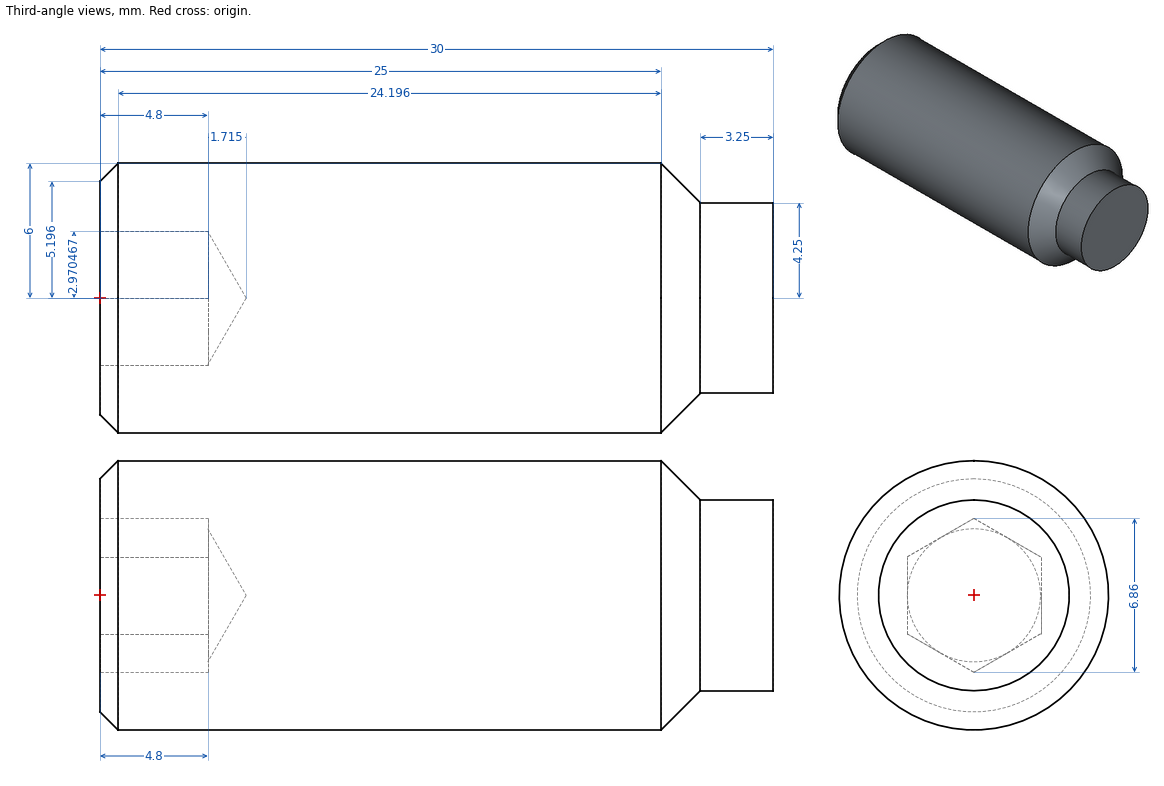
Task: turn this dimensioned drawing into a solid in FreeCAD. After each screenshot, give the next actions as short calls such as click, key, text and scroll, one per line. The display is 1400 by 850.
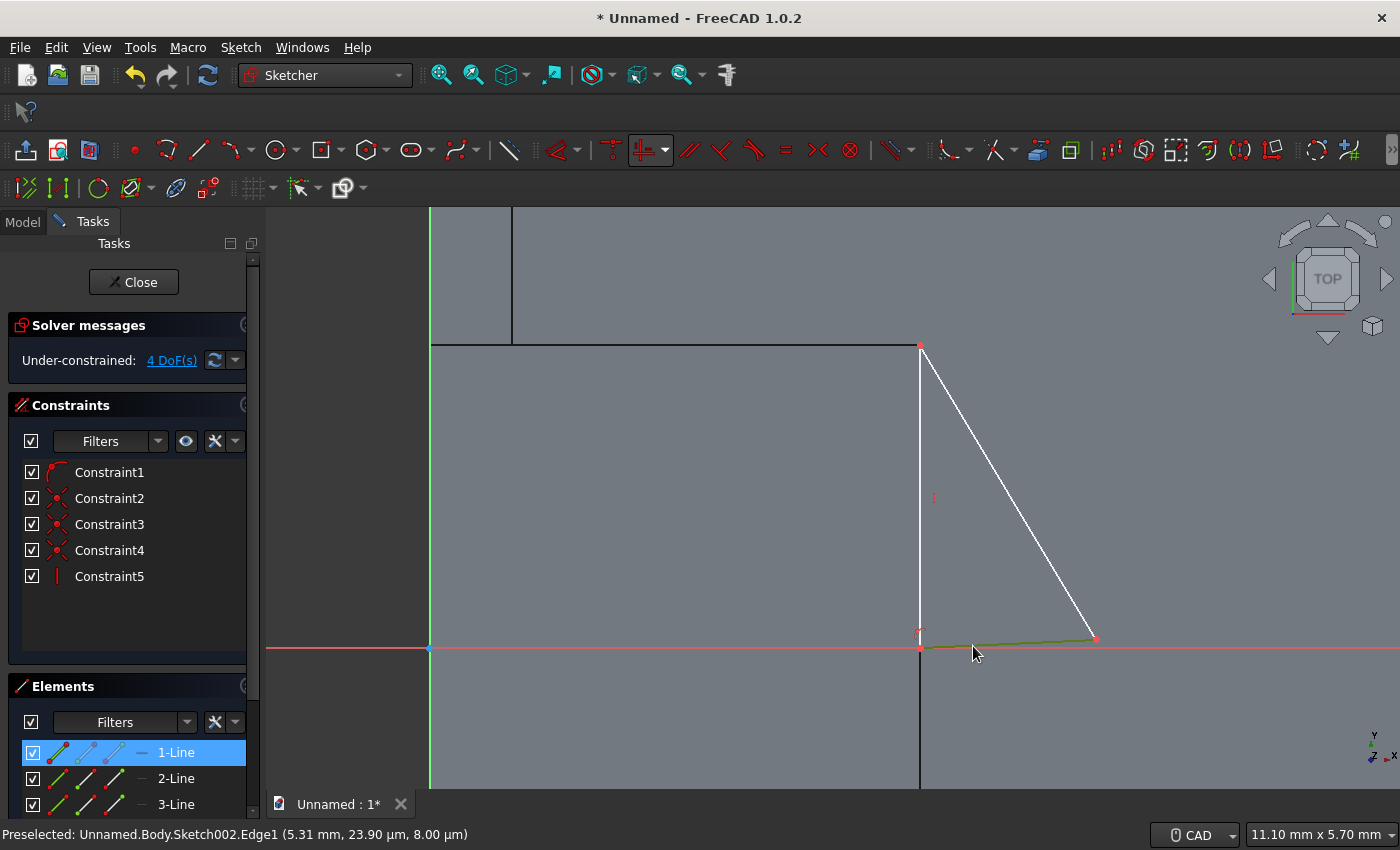
click(668, 150)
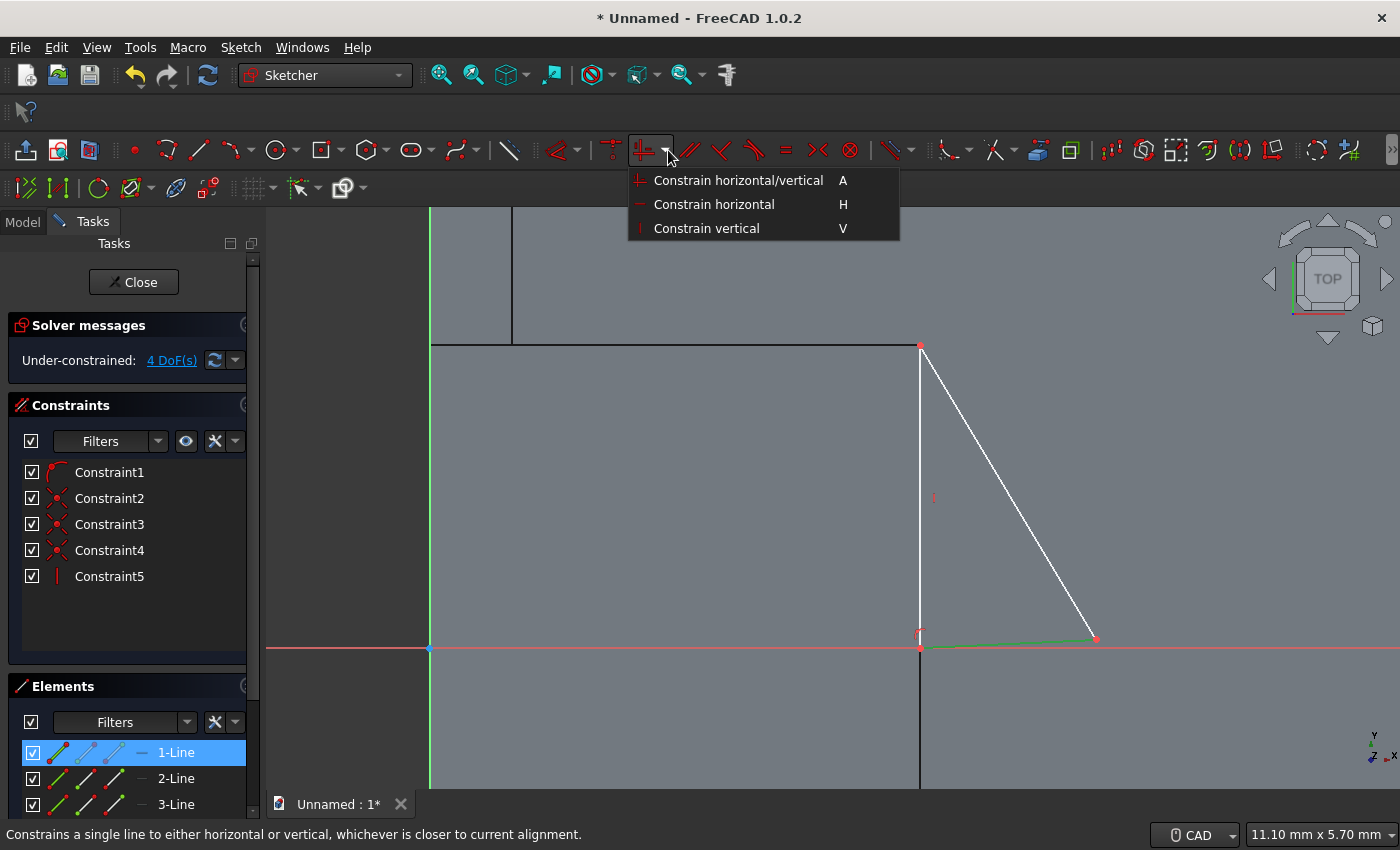
click(764, 204)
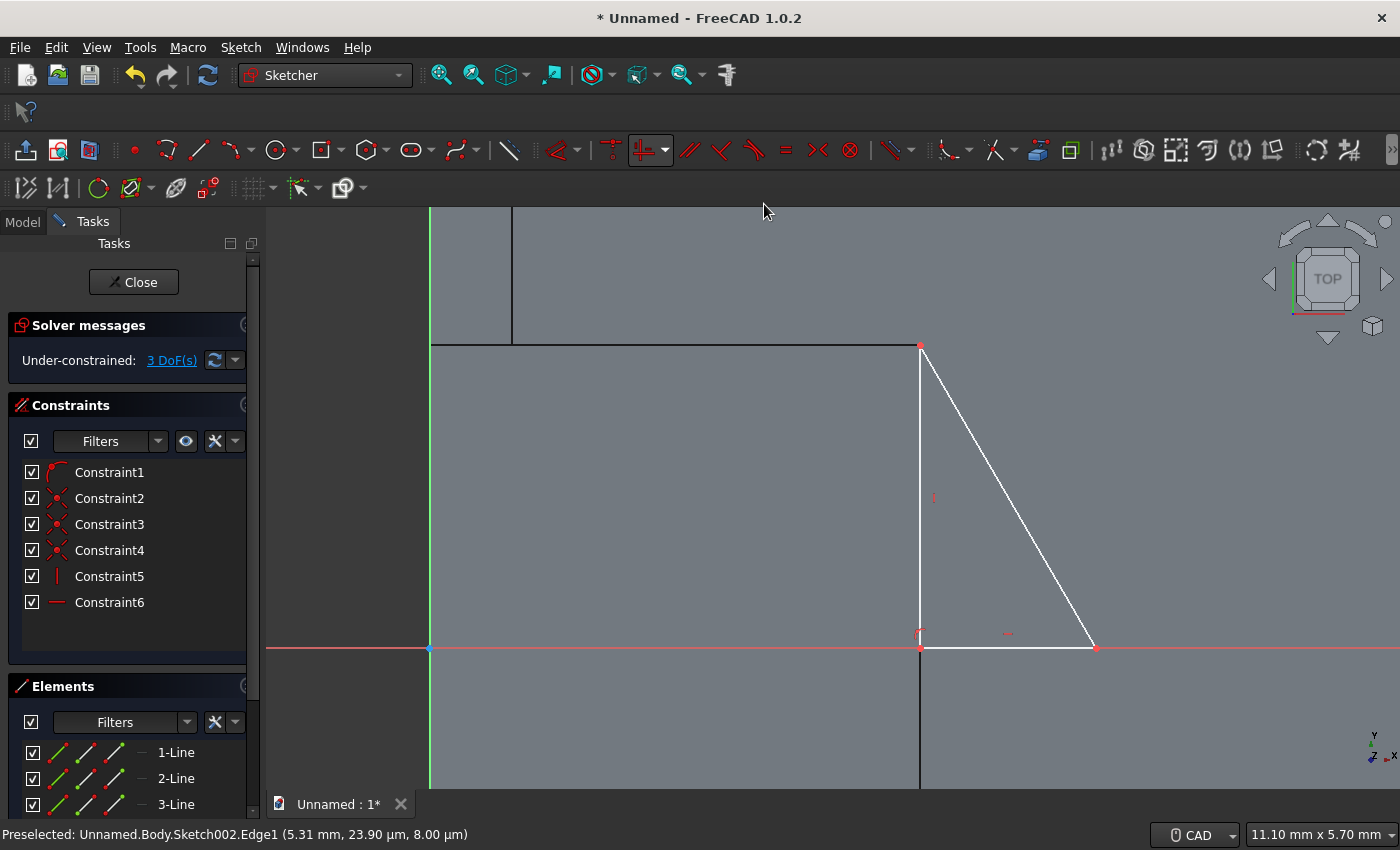
click(556, 150)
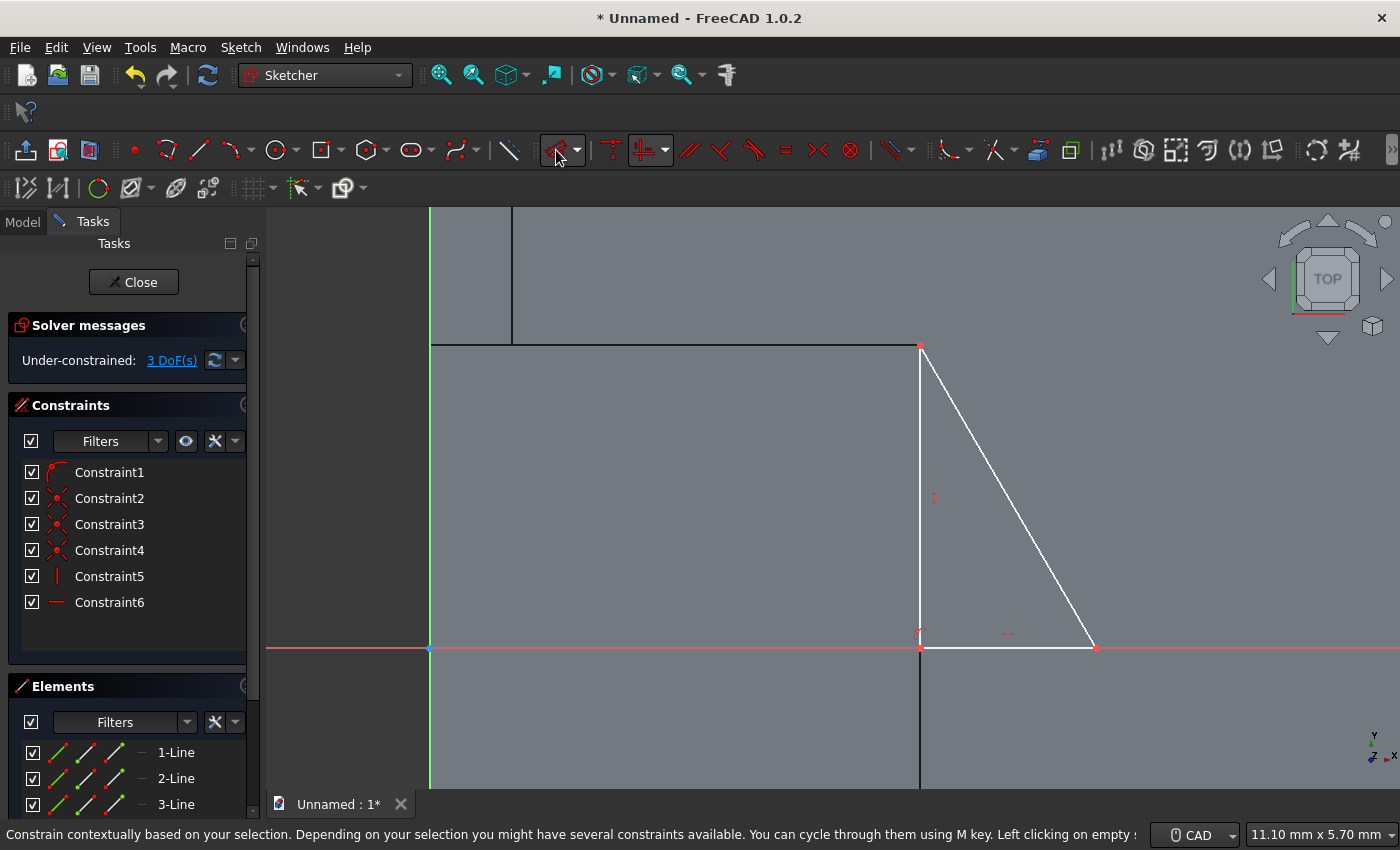
click(920, 648)
click(675, 682)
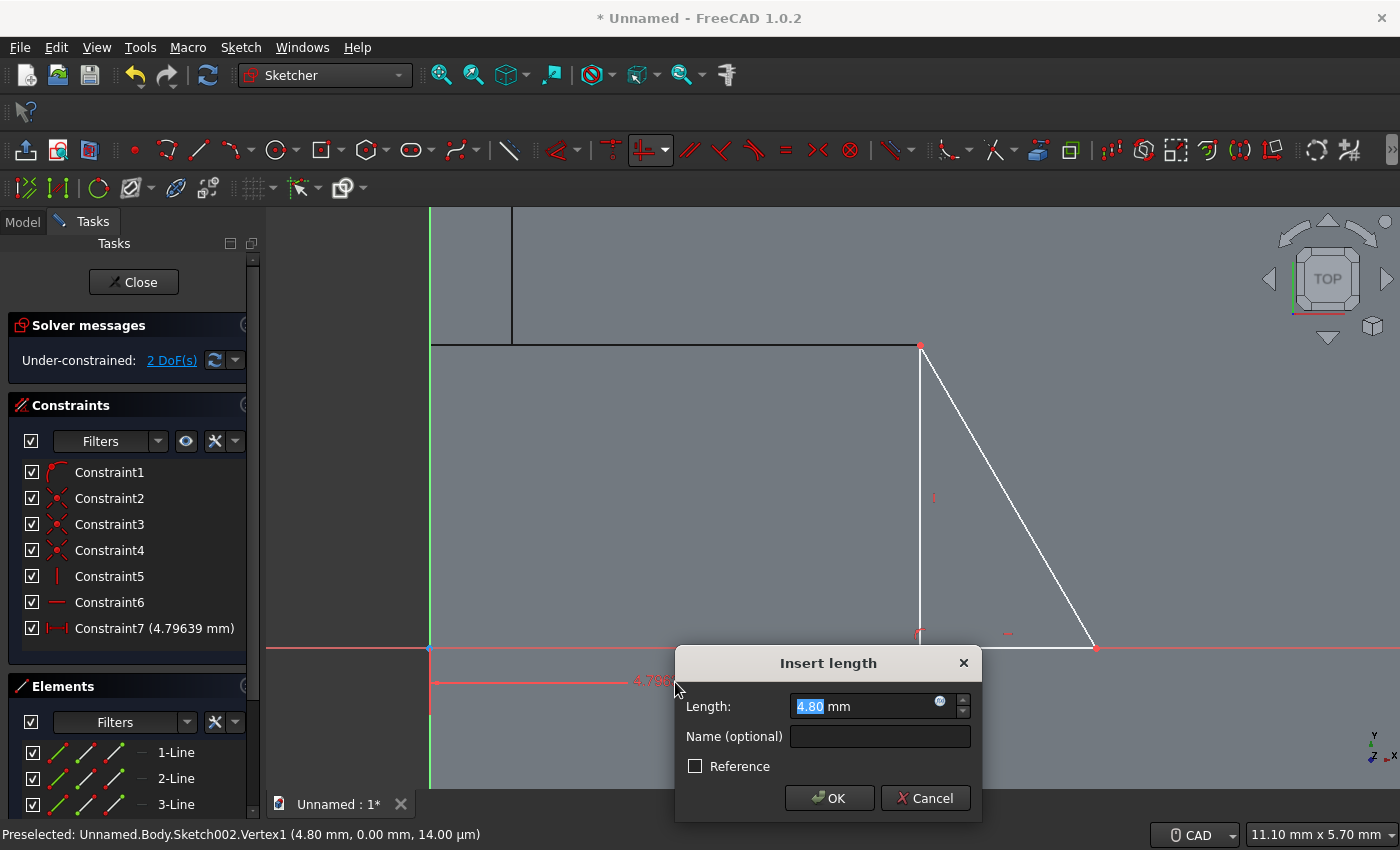
text(4.8)
key(Return)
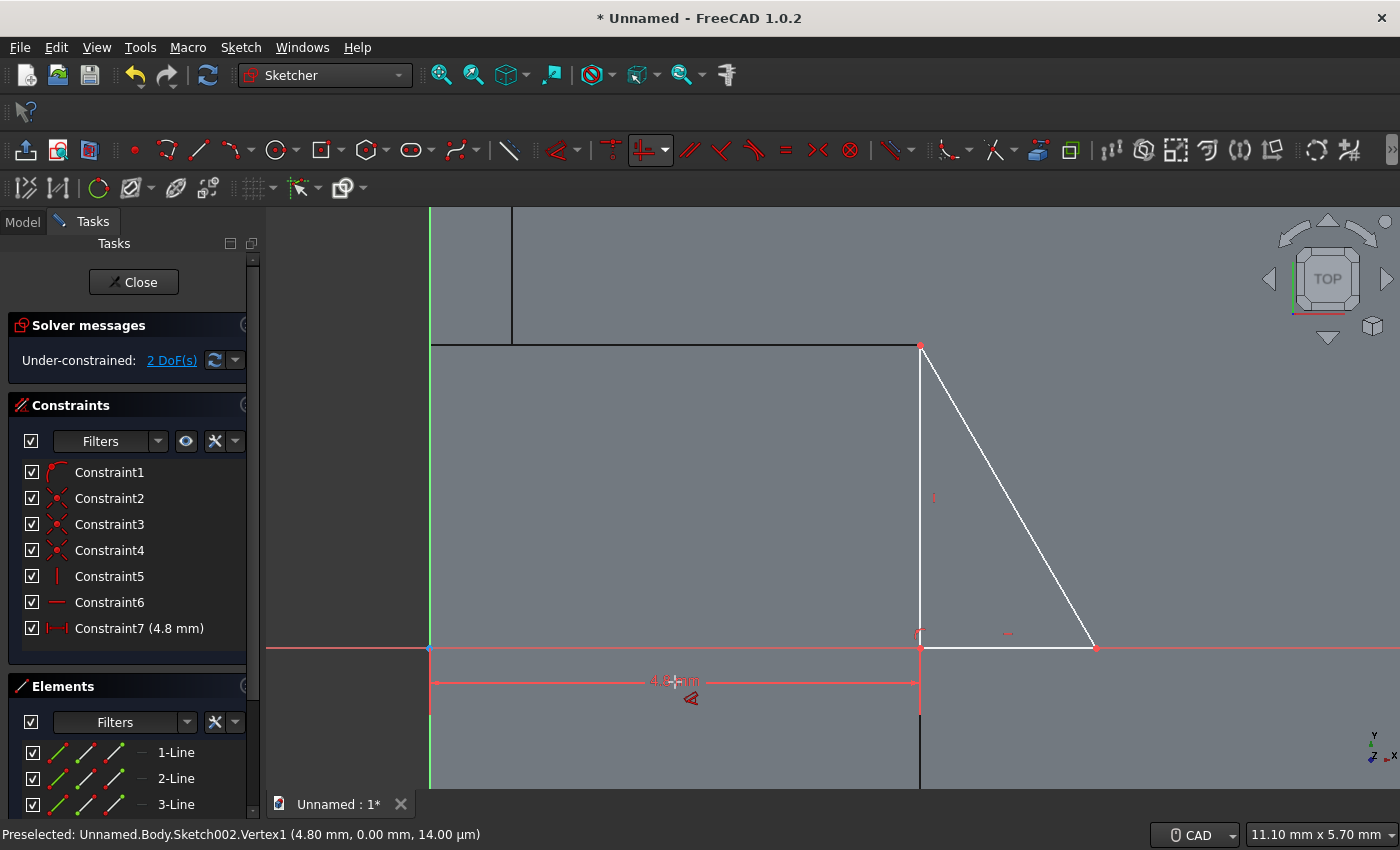
click(973, 648)
click(1008, 682)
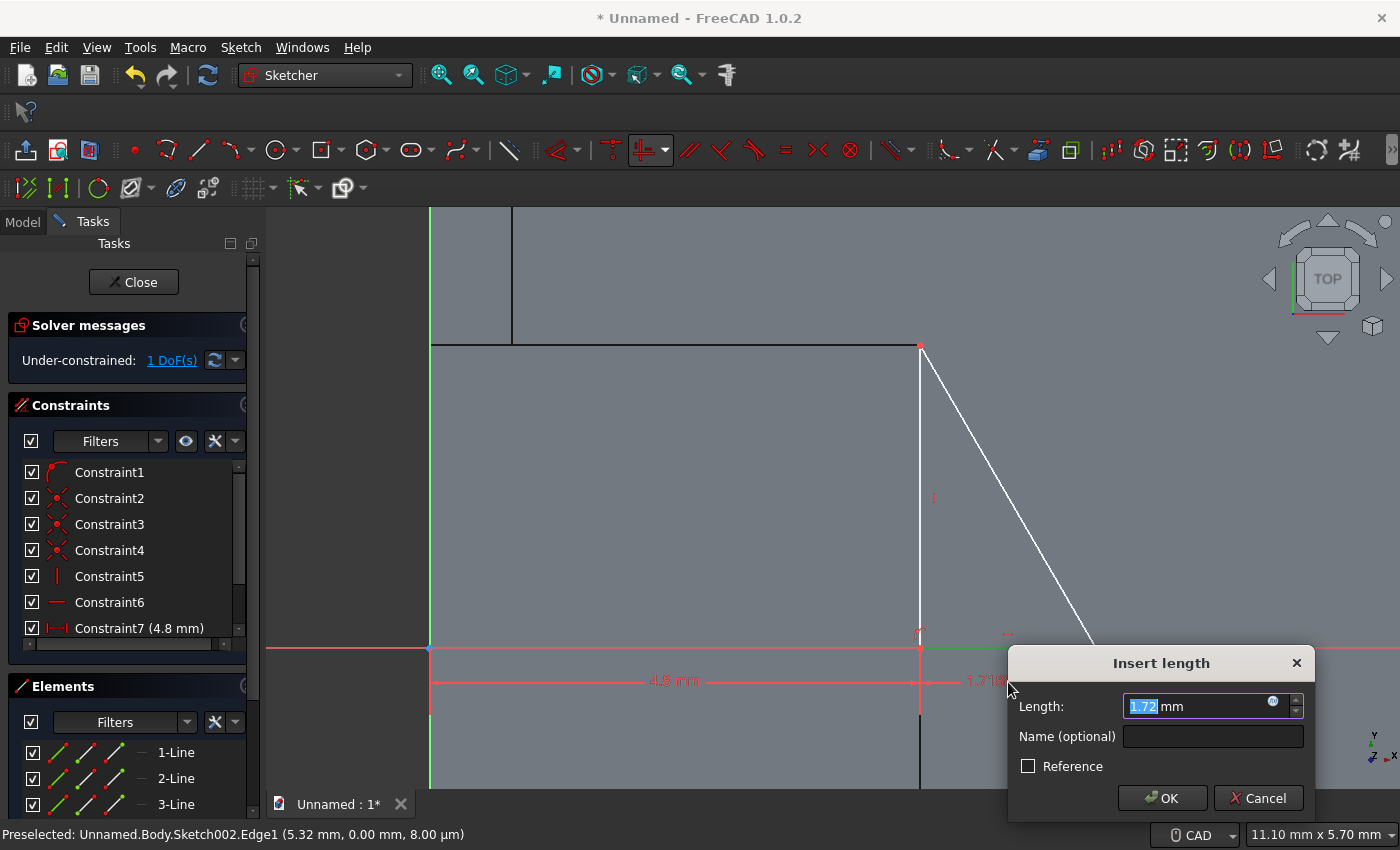
text(1.715)
key(Return)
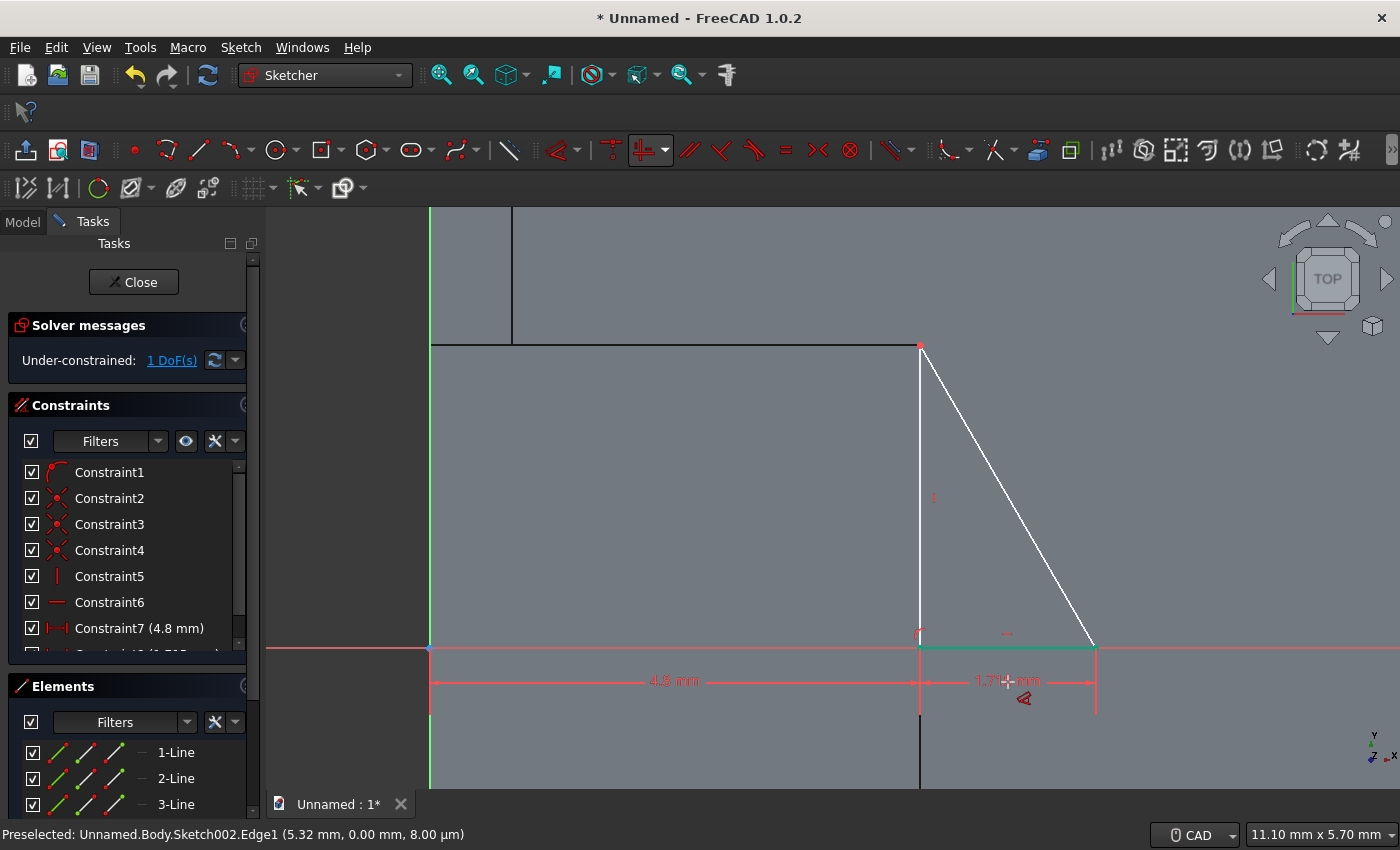
click(920, 437)
click(954, 497)